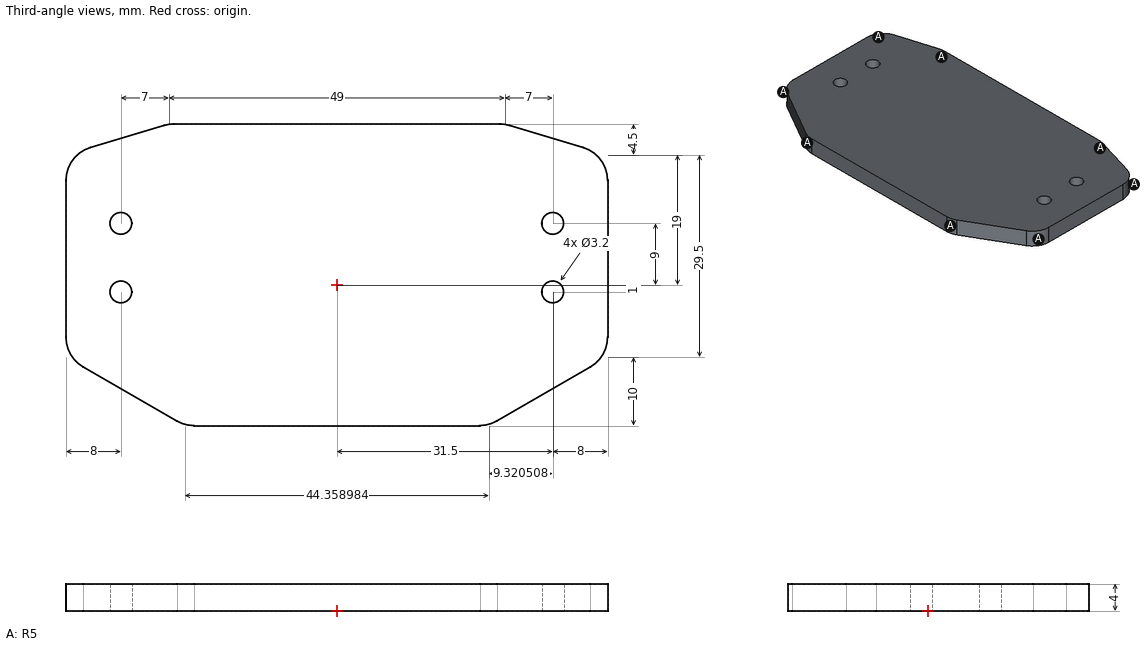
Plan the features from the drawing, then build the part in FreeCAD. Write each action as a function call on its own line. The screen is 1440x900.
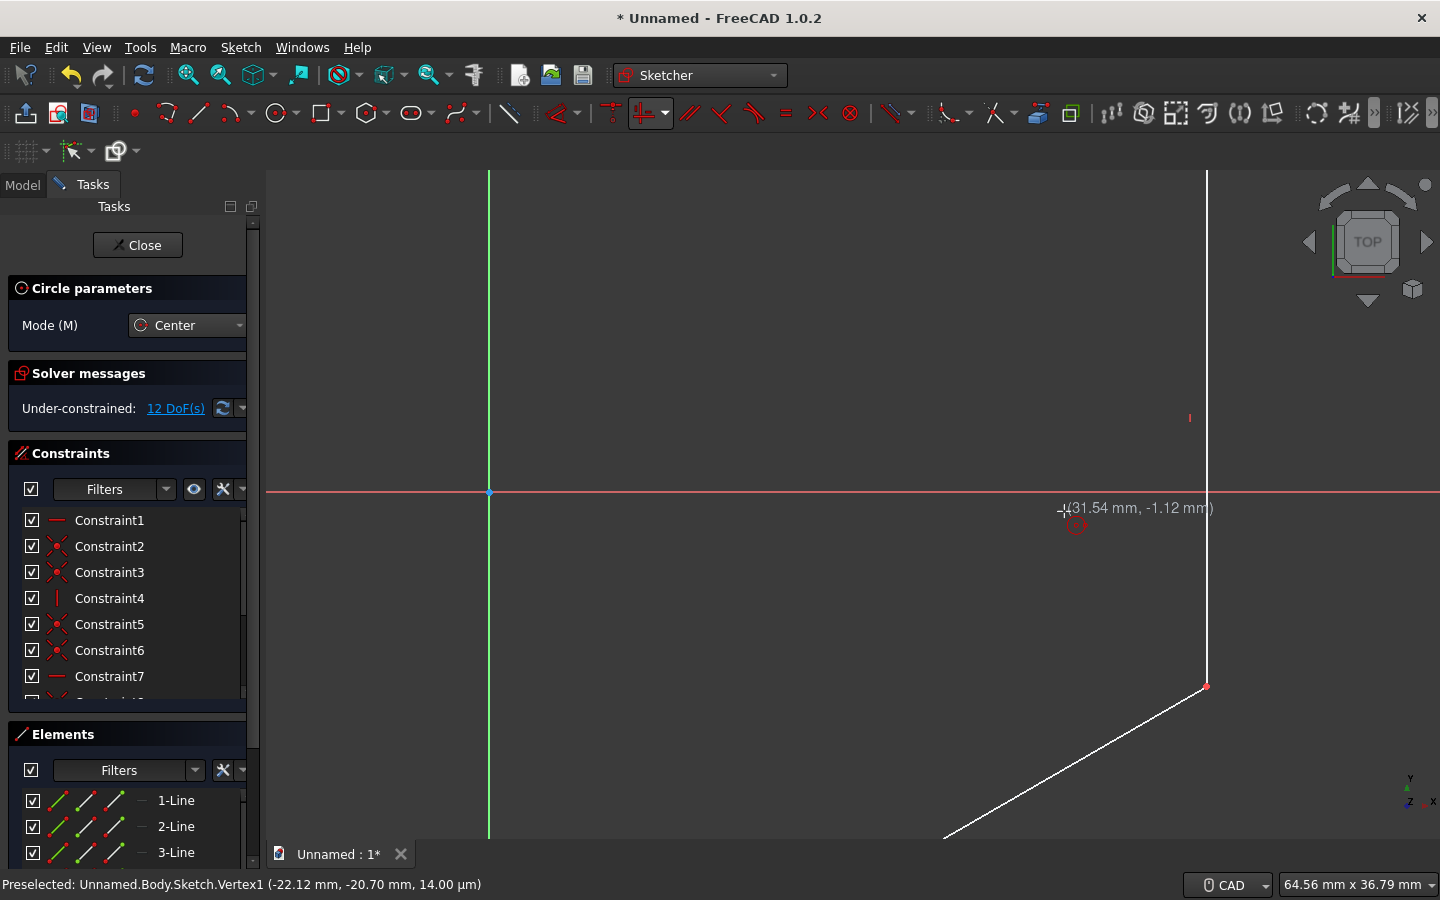
click(1062, 511)
move(1083, 531)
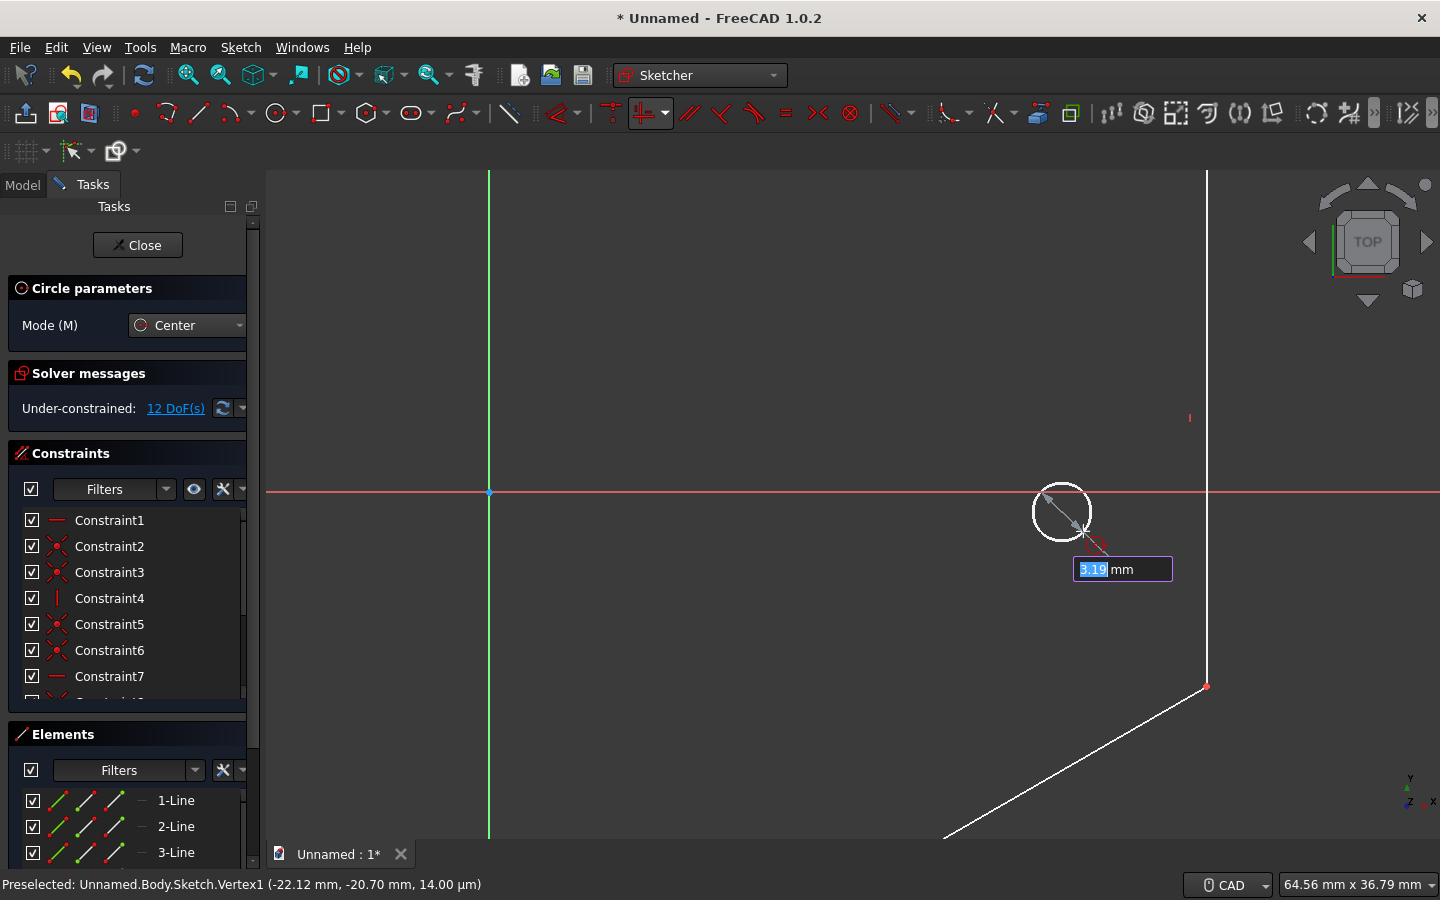
text(3.2)
key(Return)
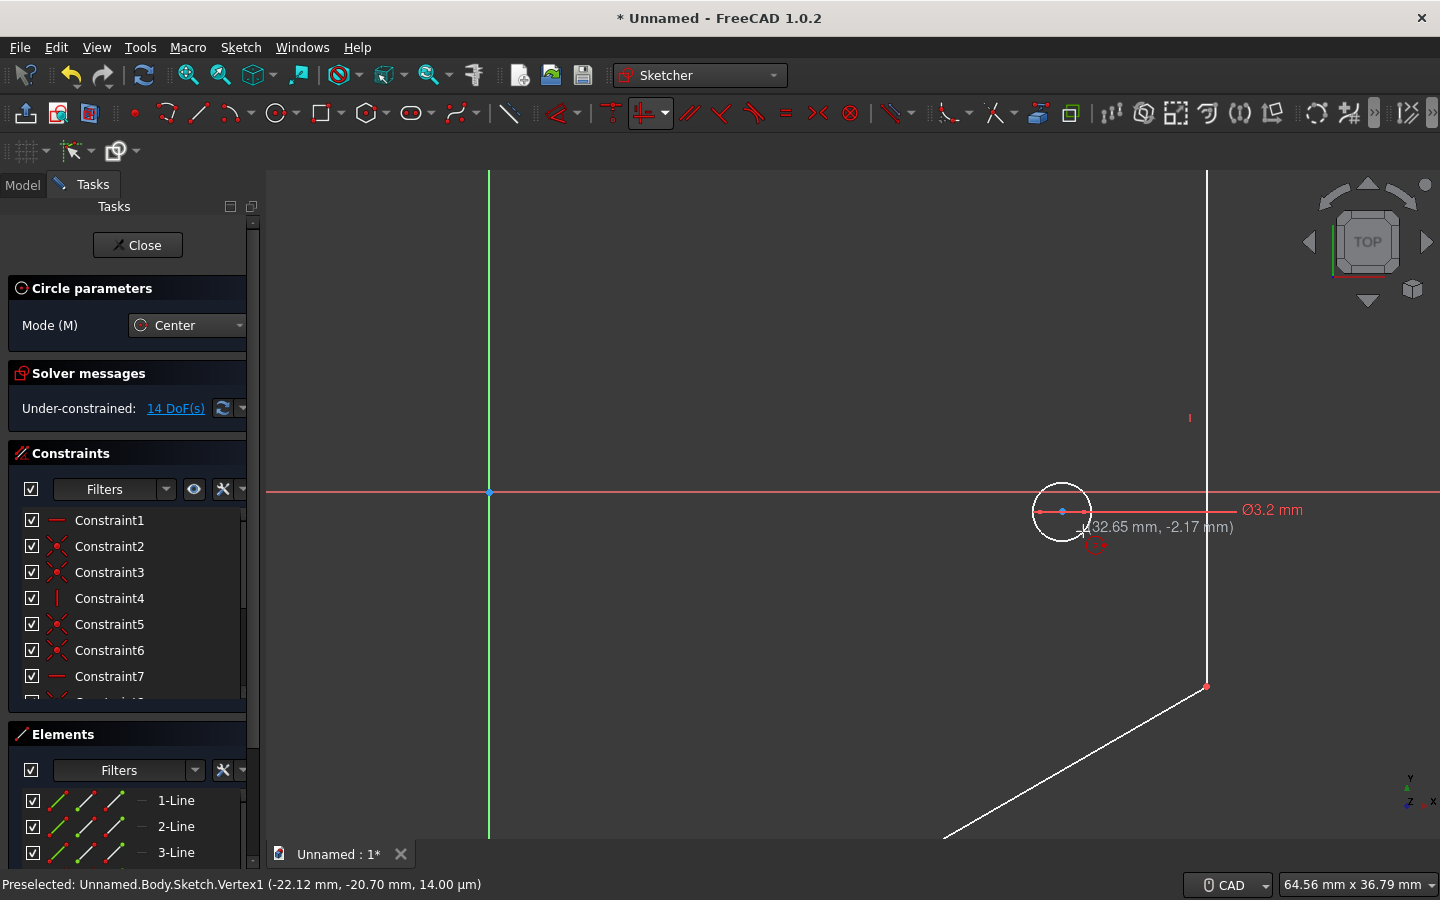
scroll(1025, 537, down, 4)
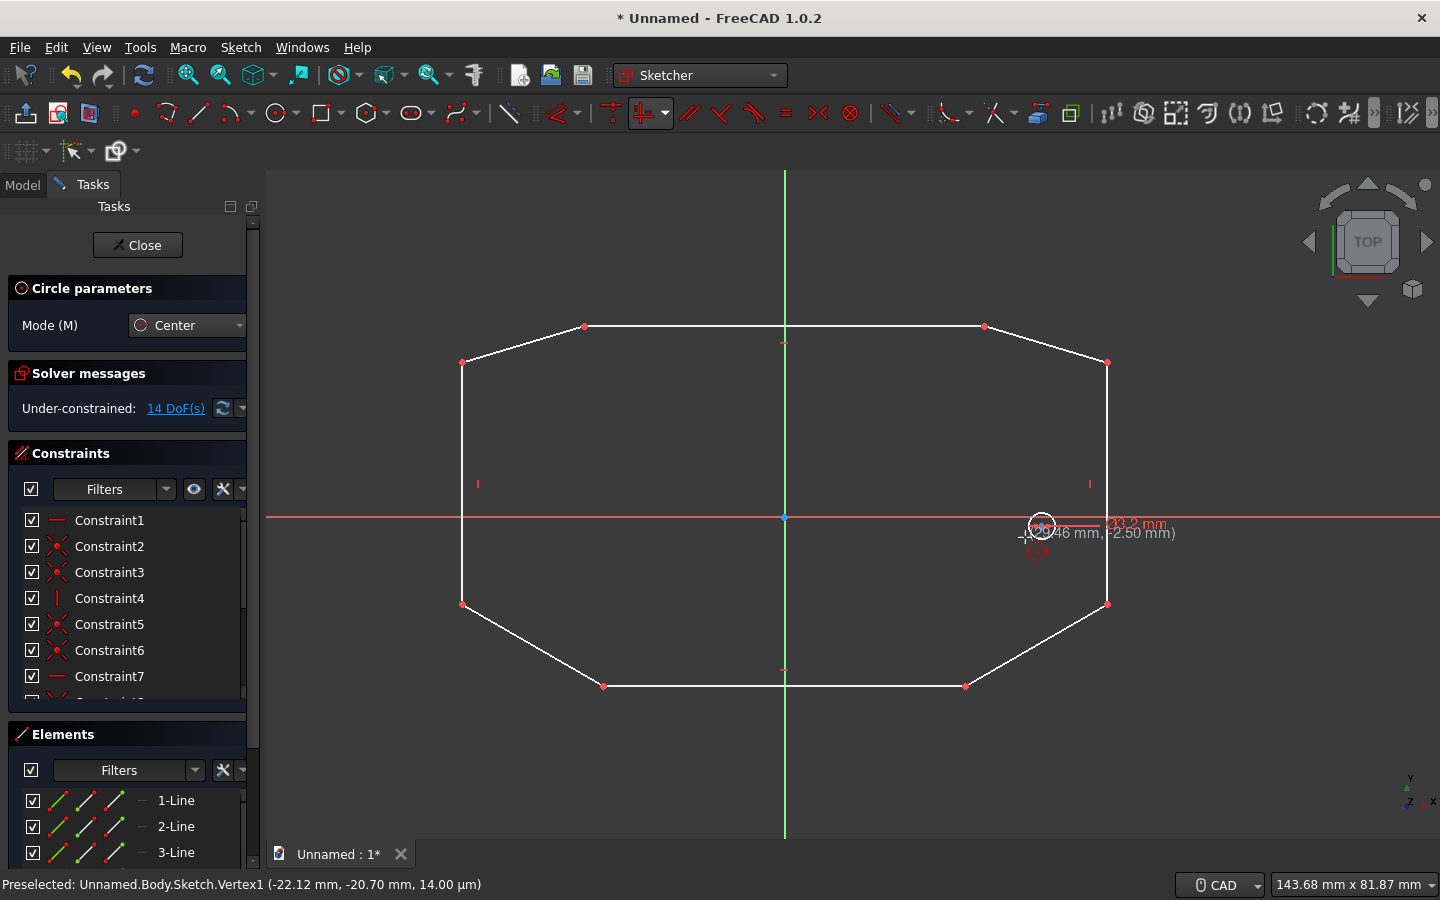
scroll(527, 525, up, 4)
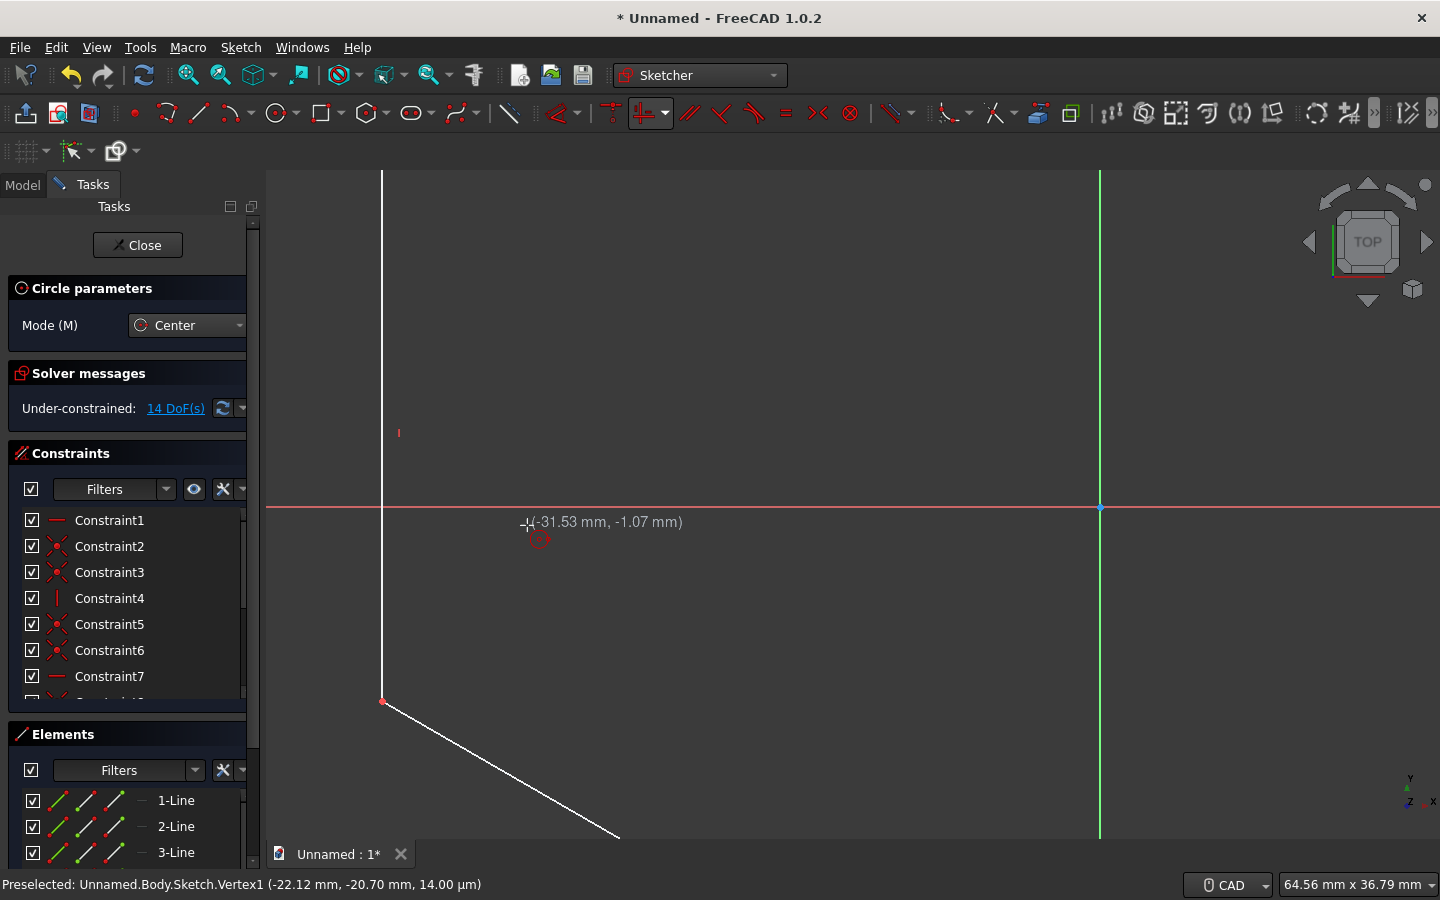
click(527, 525)
move(548, 546)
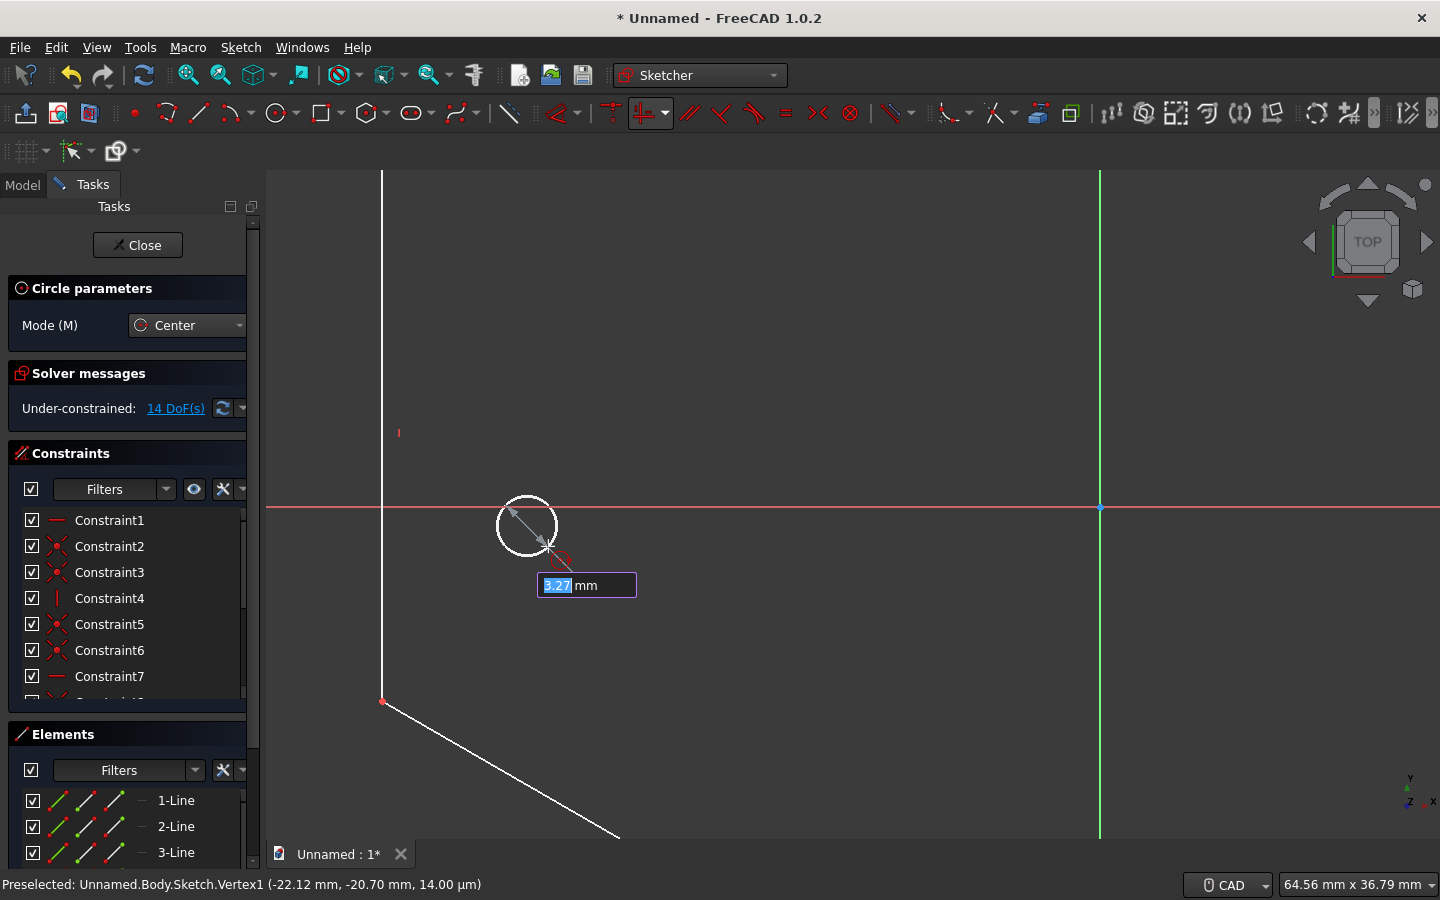
text(3.2)
key(Return)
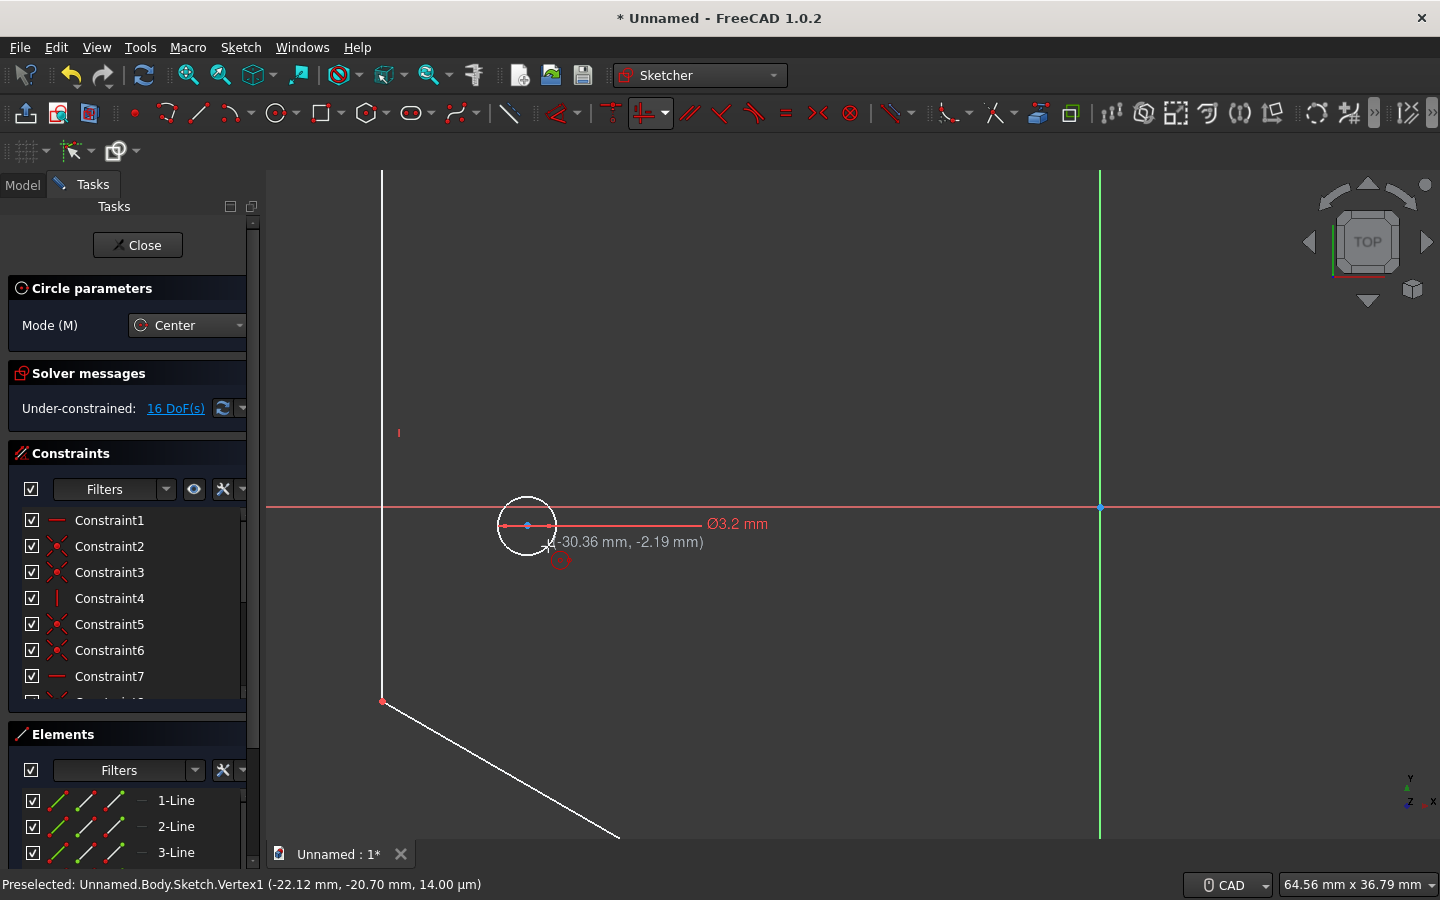
scroll(527, 525, down, 4)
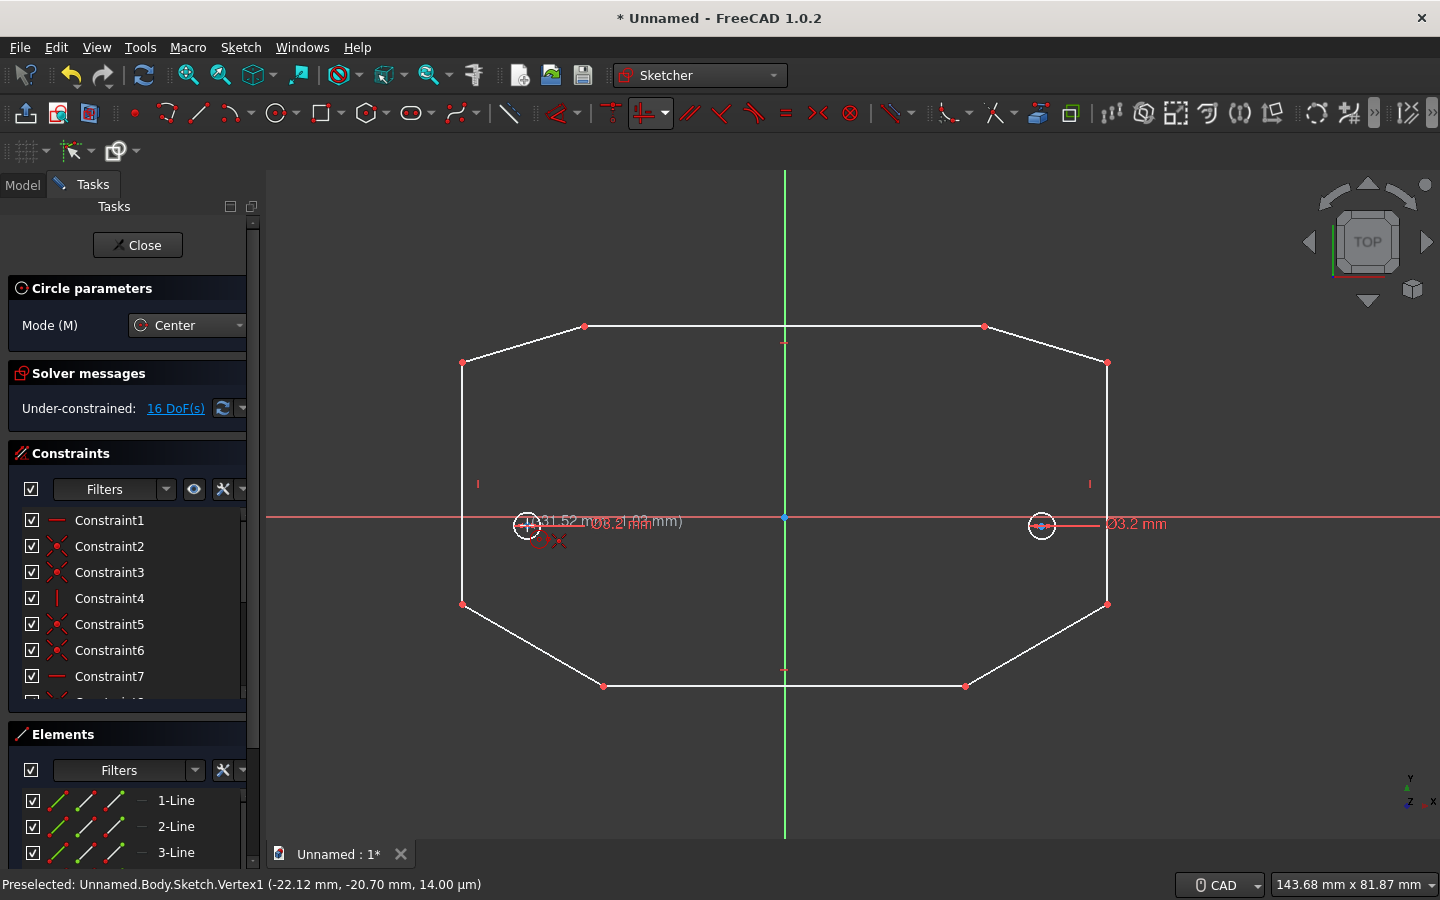
scroll(1042, 444, up, 3)